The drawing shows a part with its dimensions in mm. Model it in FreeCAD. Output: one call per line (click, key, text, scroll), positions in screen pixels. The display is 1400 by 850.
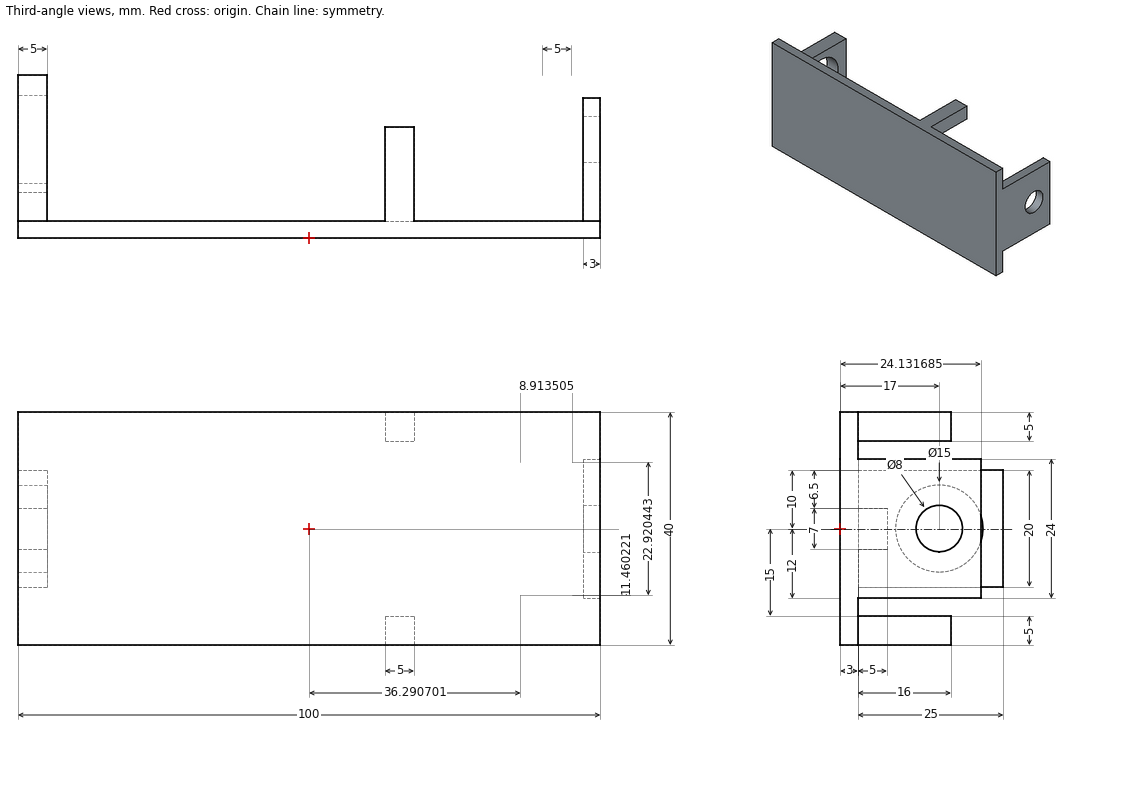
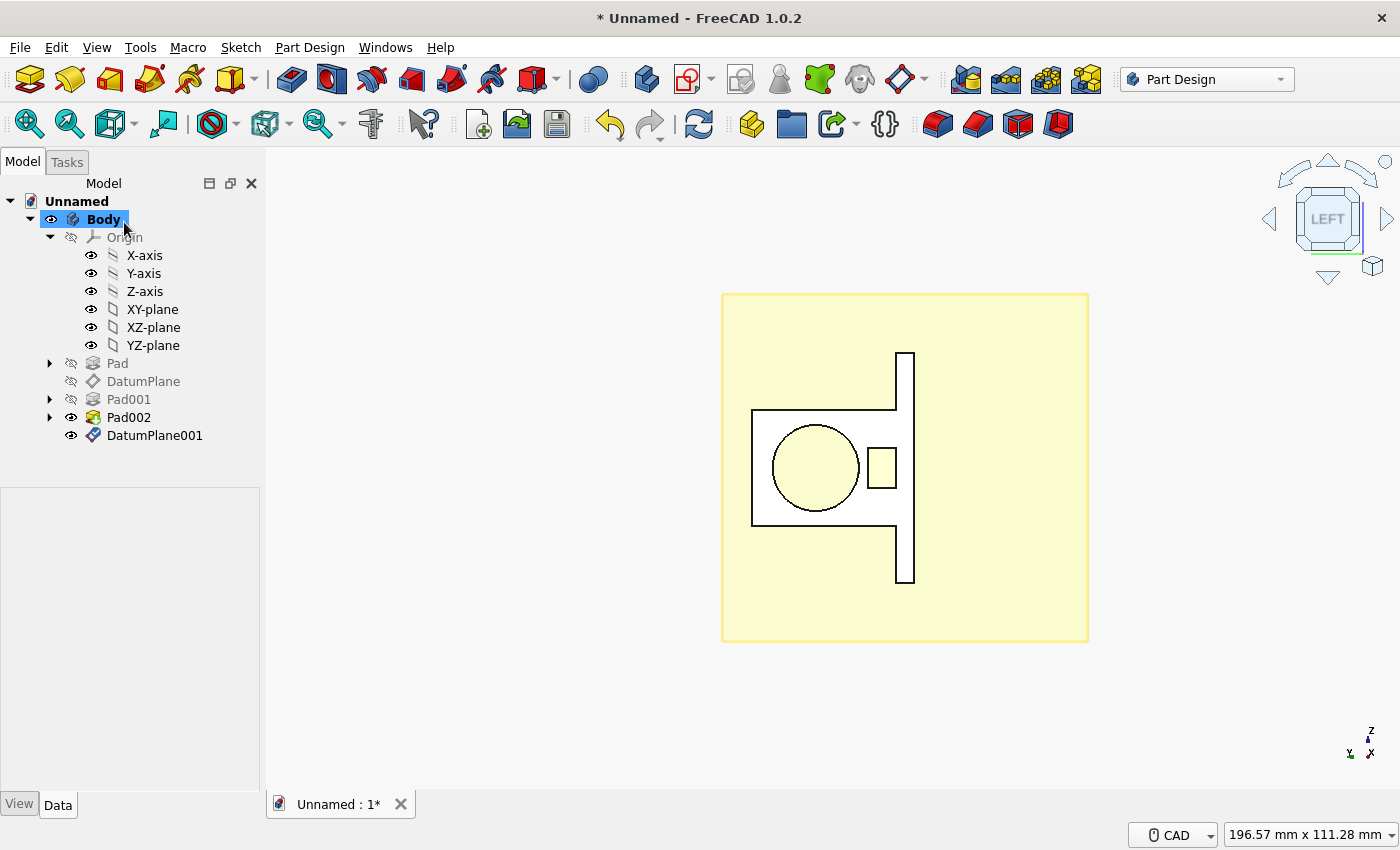
click(116, 435)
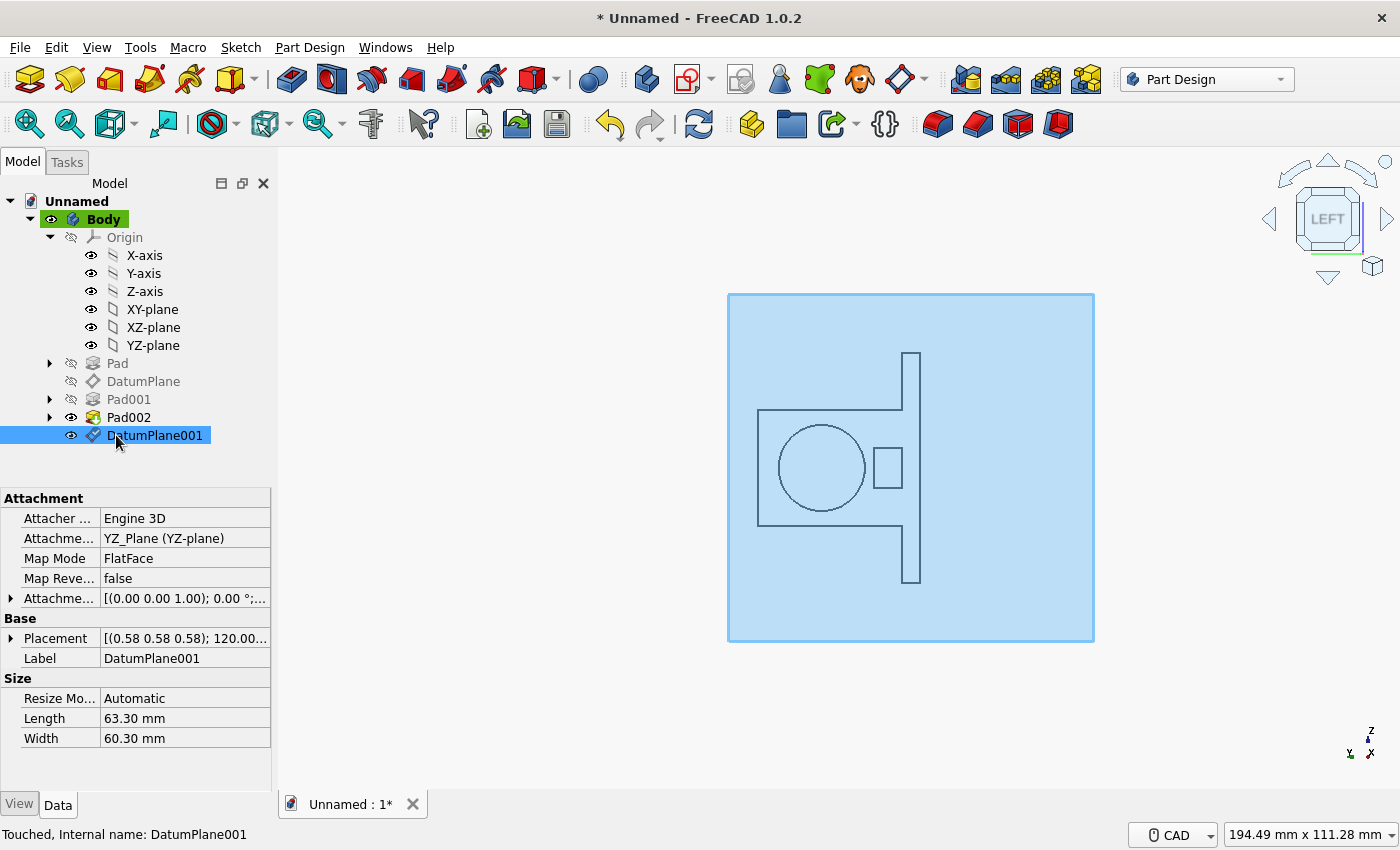
click(688, 80)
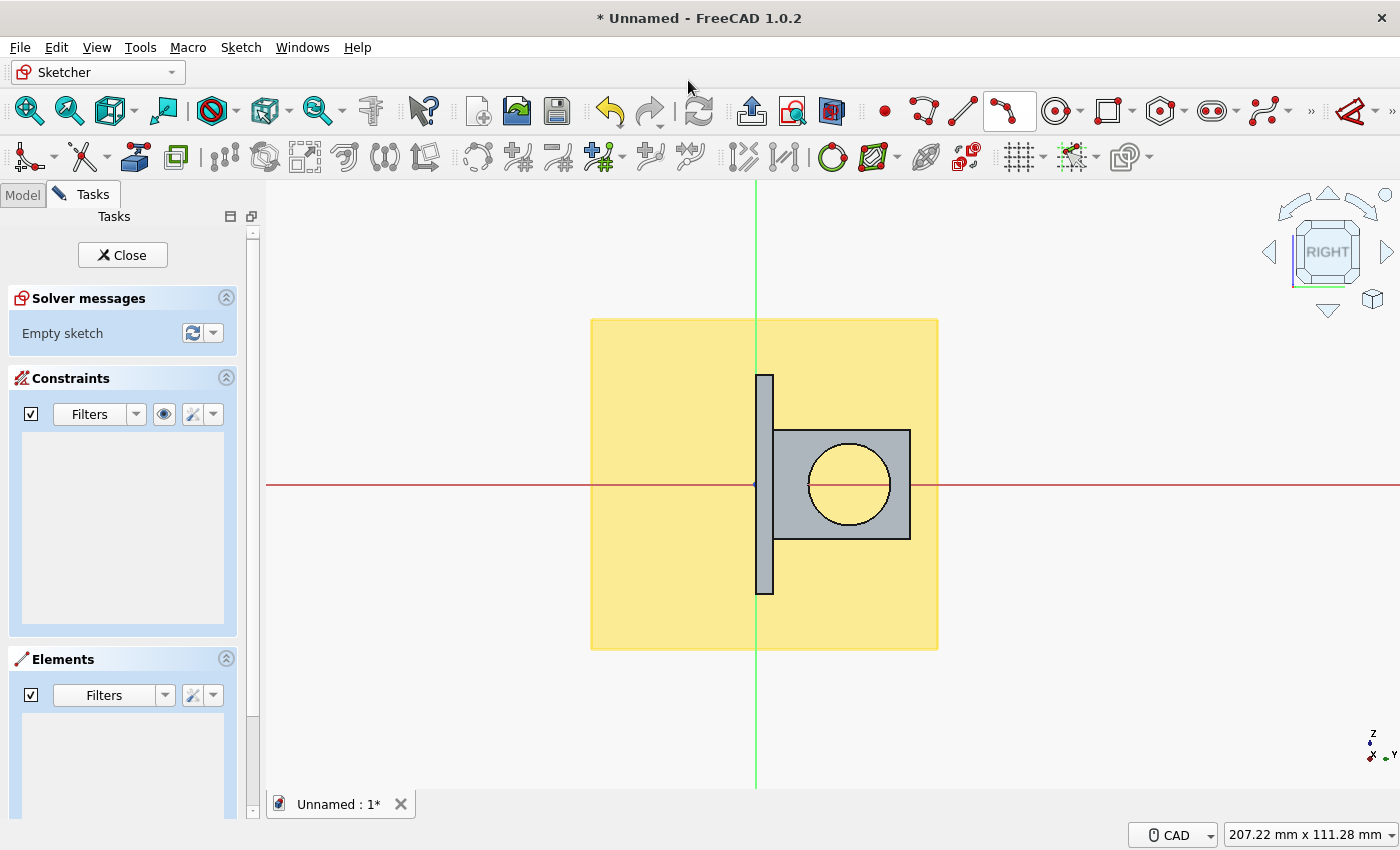
key(q)
key(s)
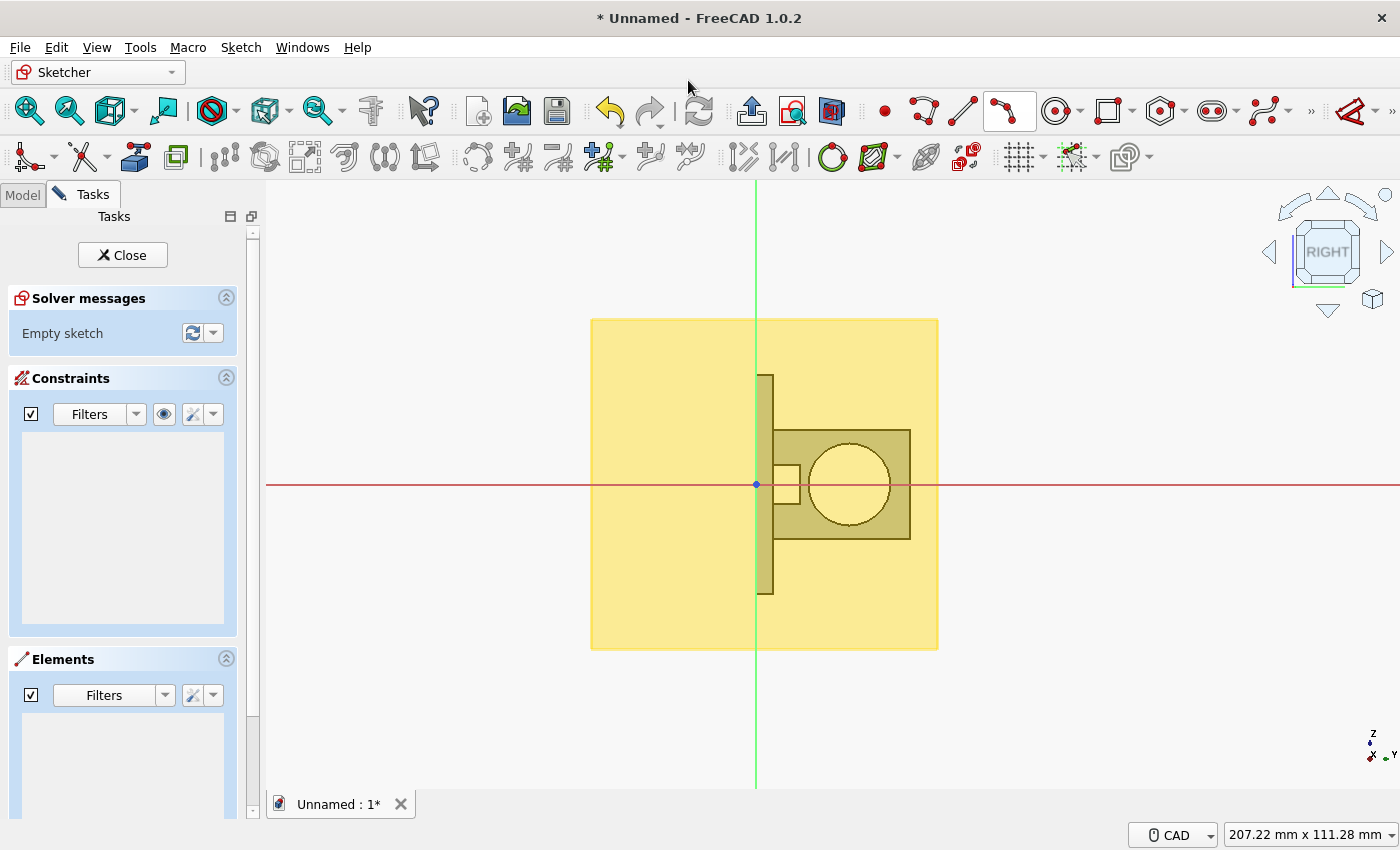
scroll(862, 485, up, 3)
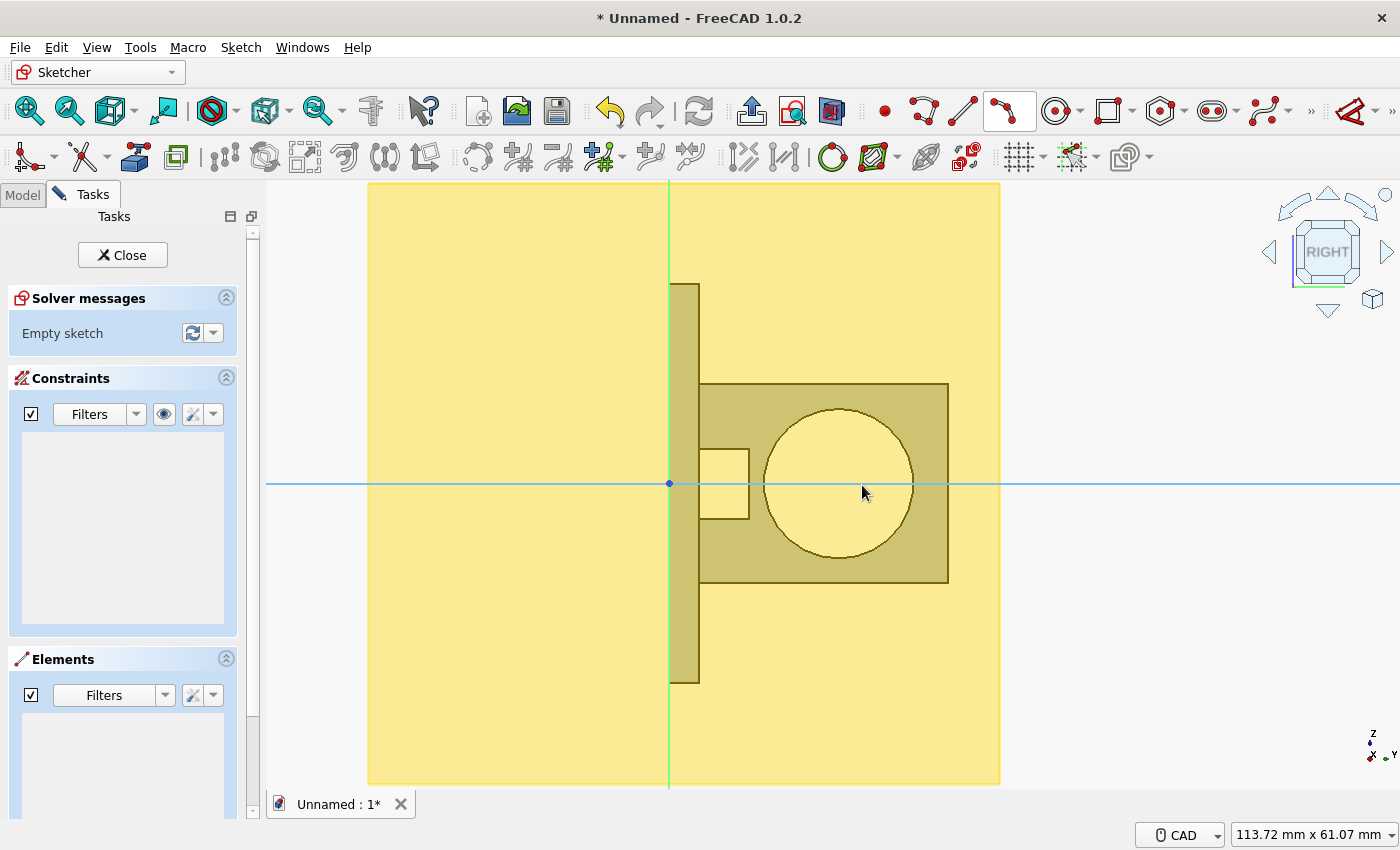
click(1108, 112)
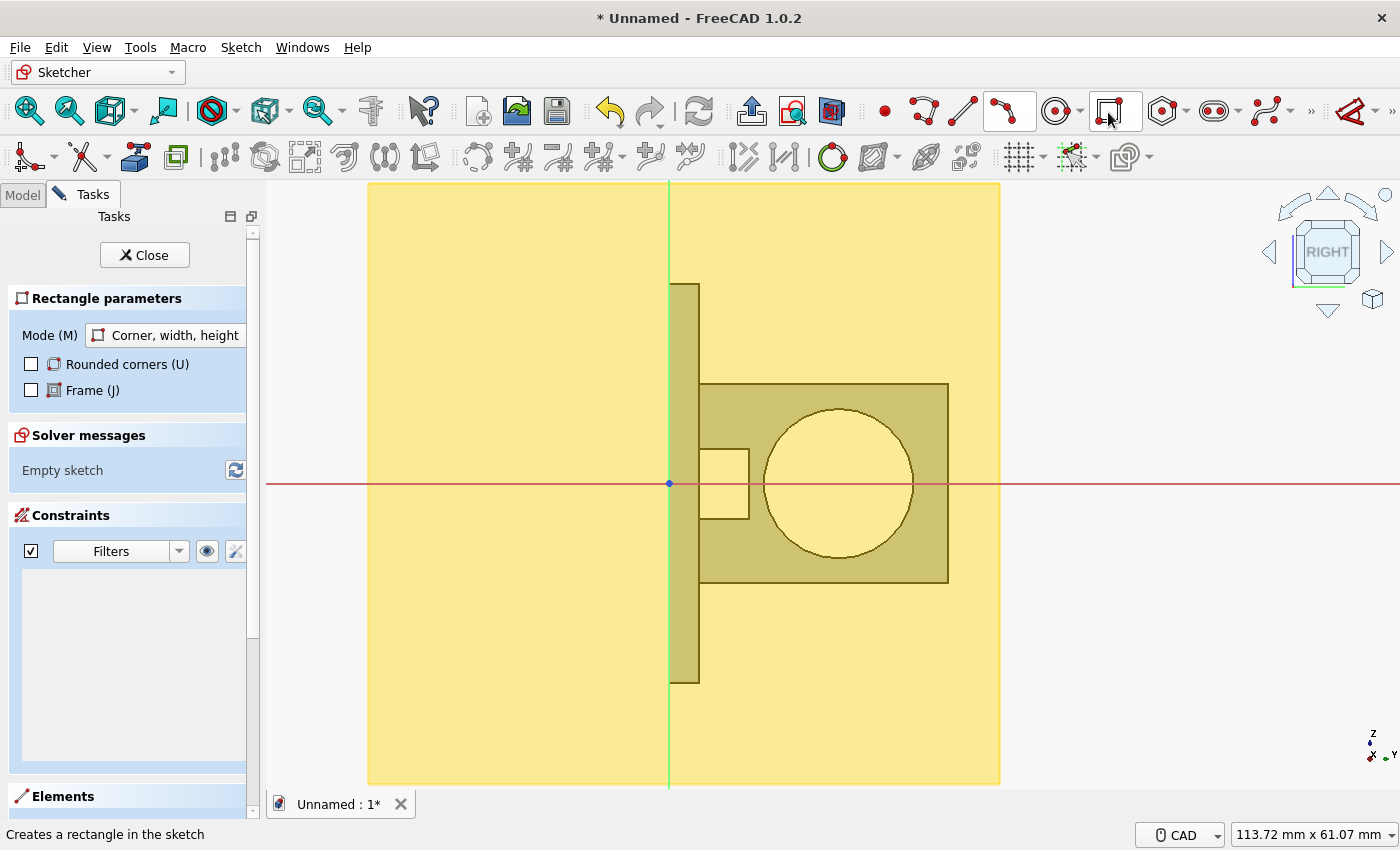
click(699, 633)
move(859, 683)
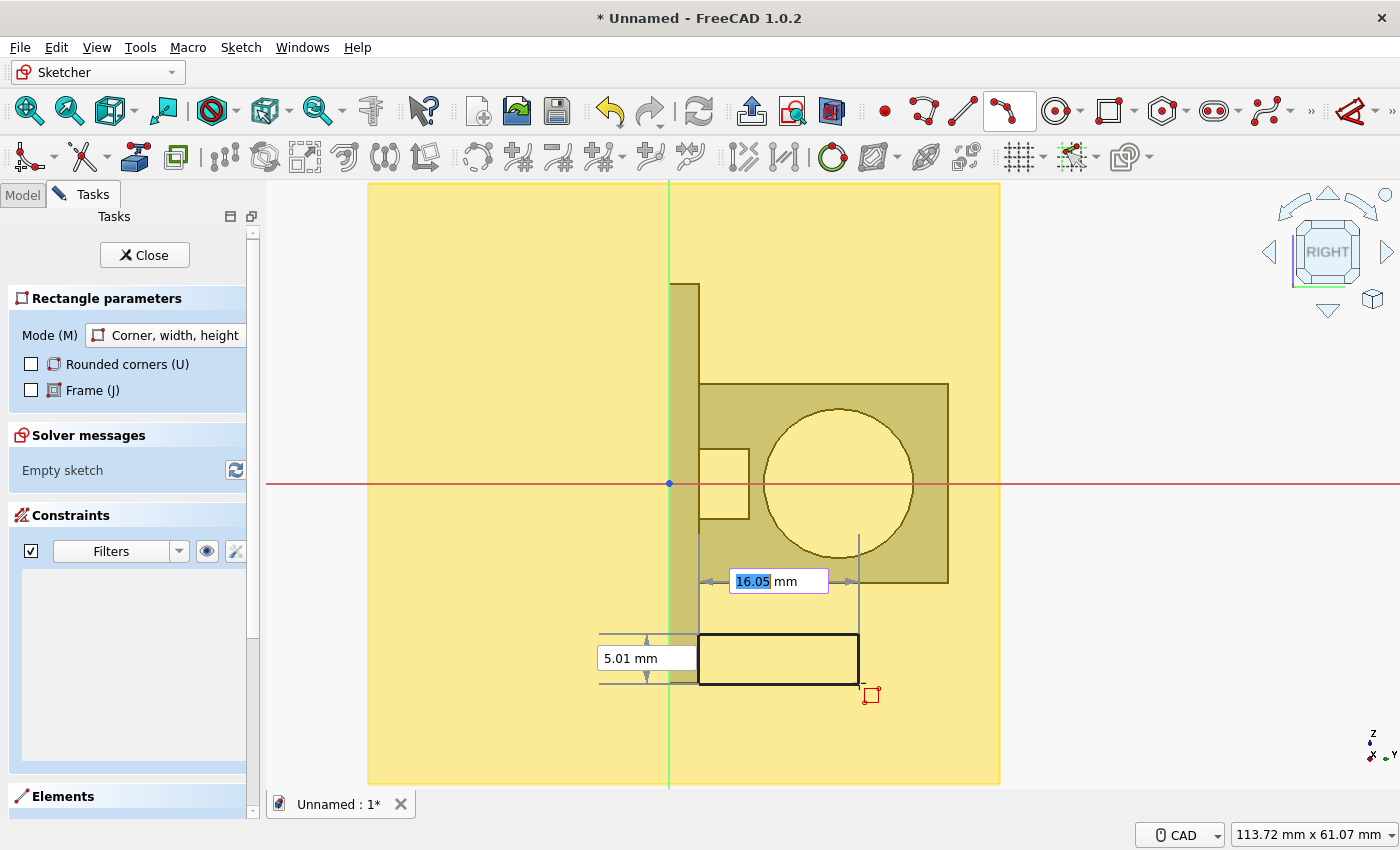
text(16)
key(Tab)
text(5)
key(Return)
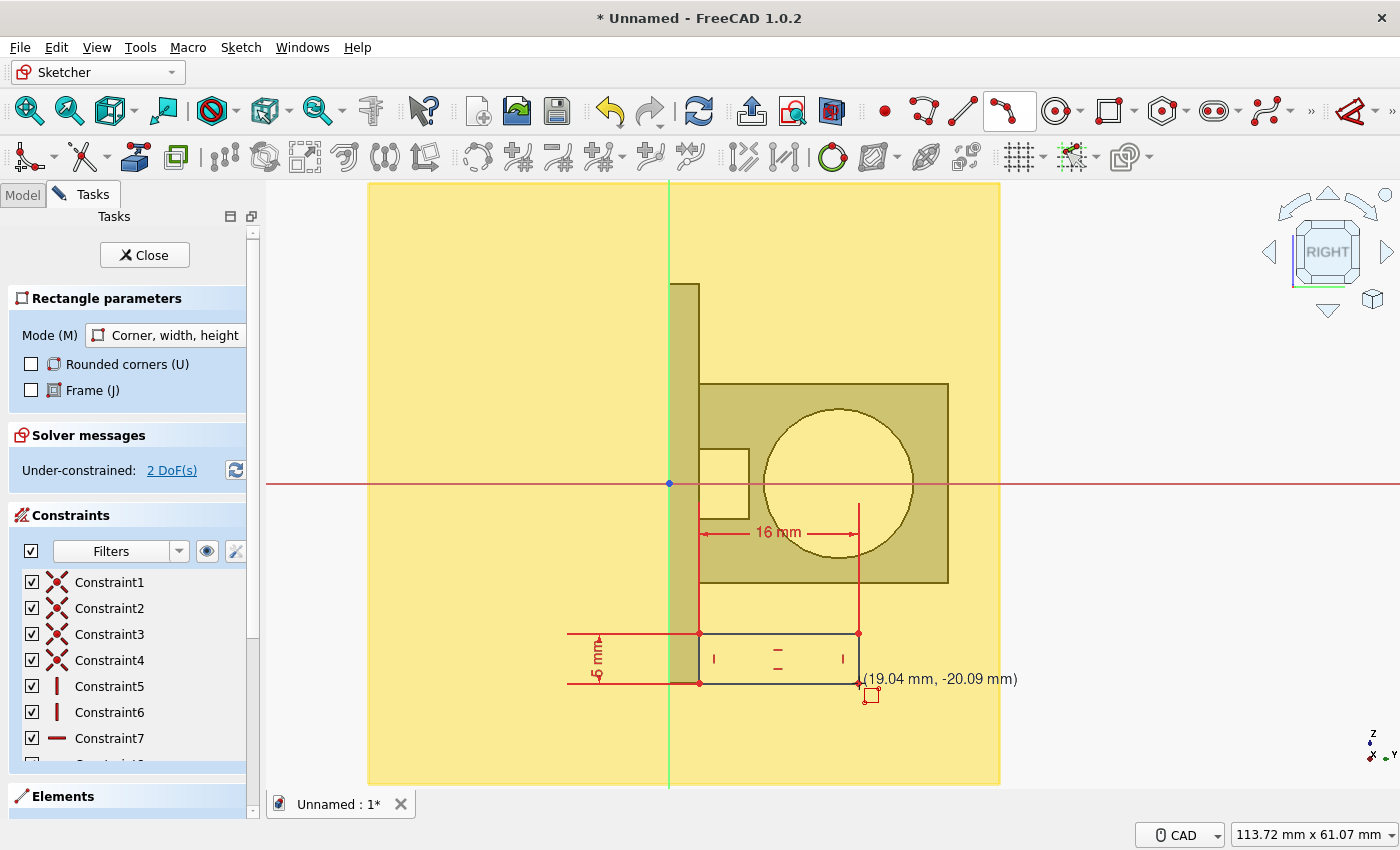
click(699, 284)
move(859, 334)